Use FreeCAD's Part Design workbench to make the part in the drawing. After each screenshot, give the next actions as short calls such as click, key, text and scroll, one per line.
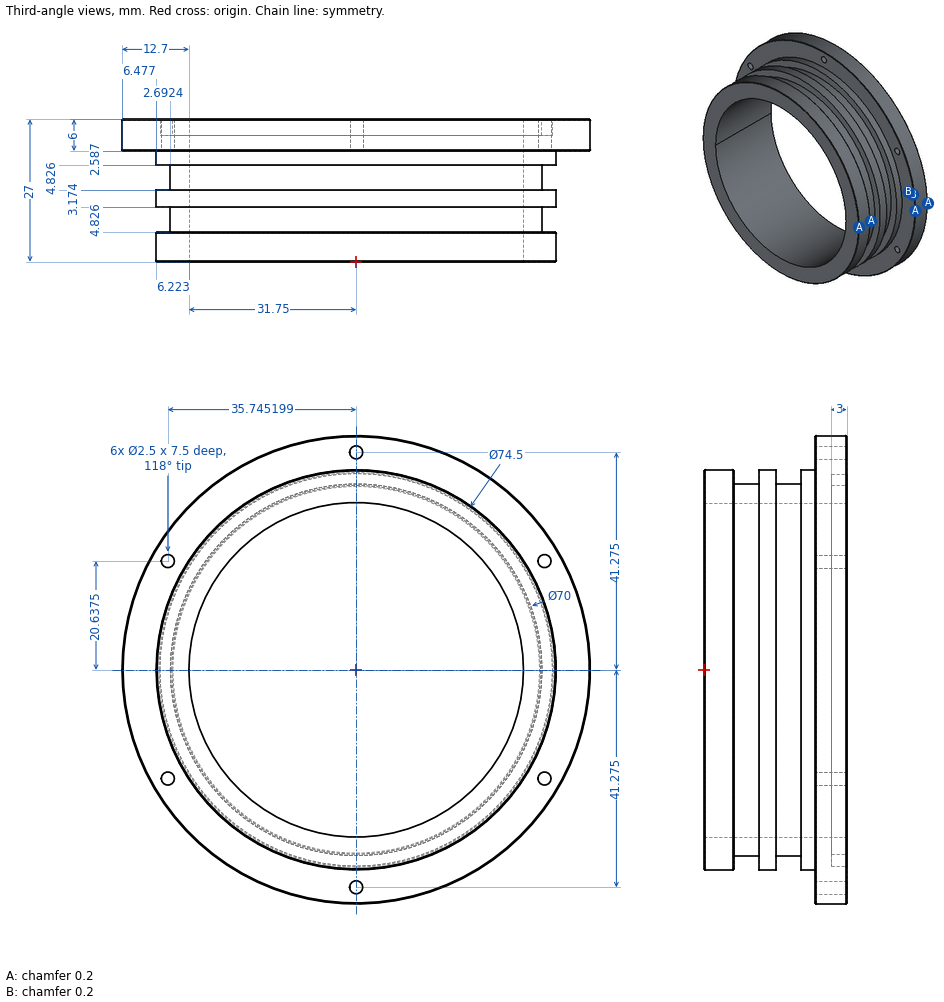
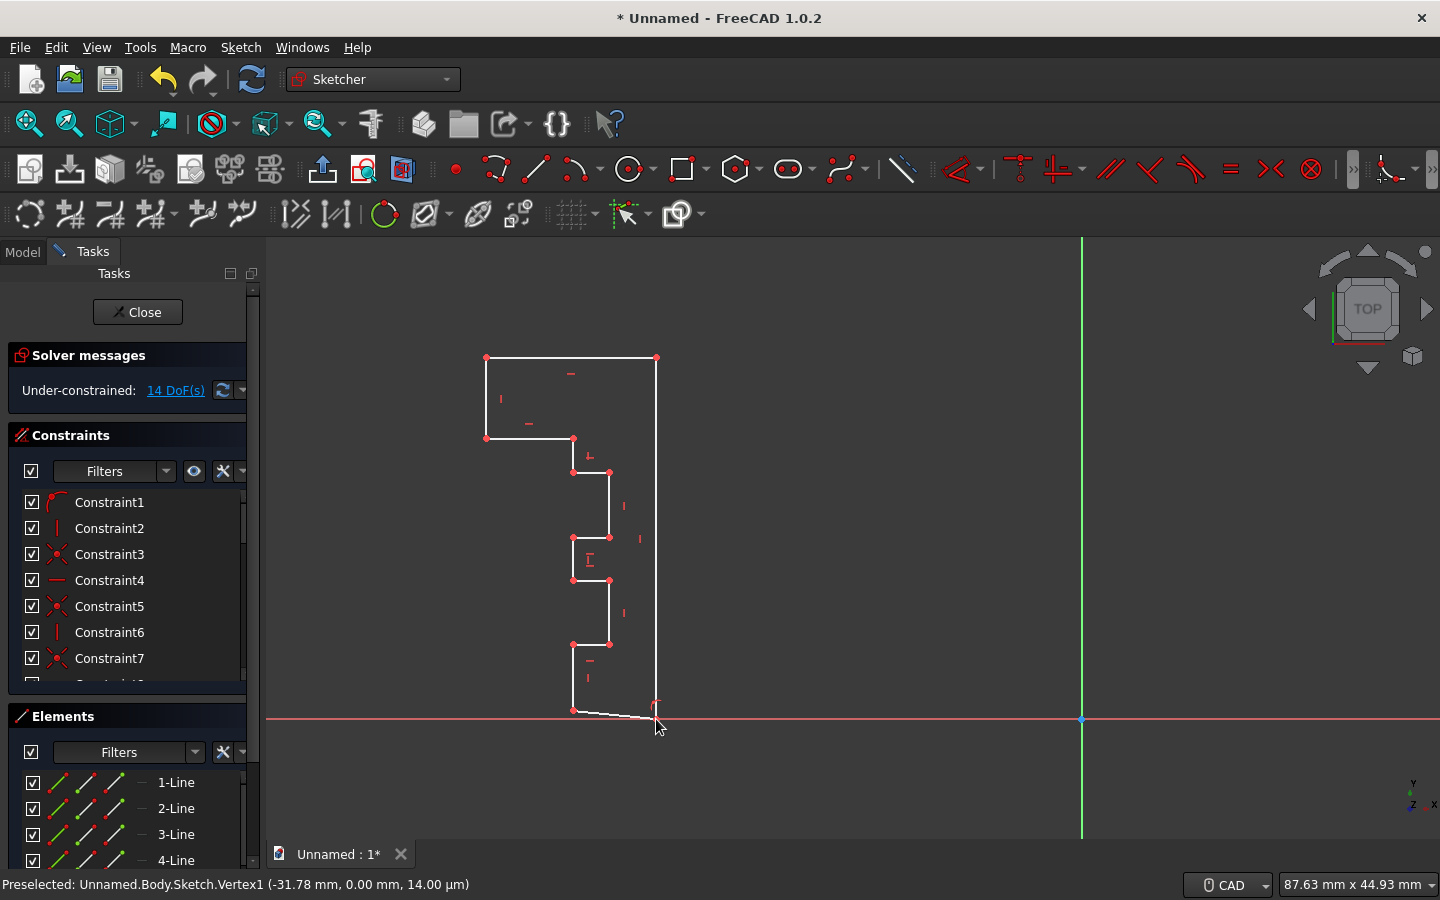
click(631, 717)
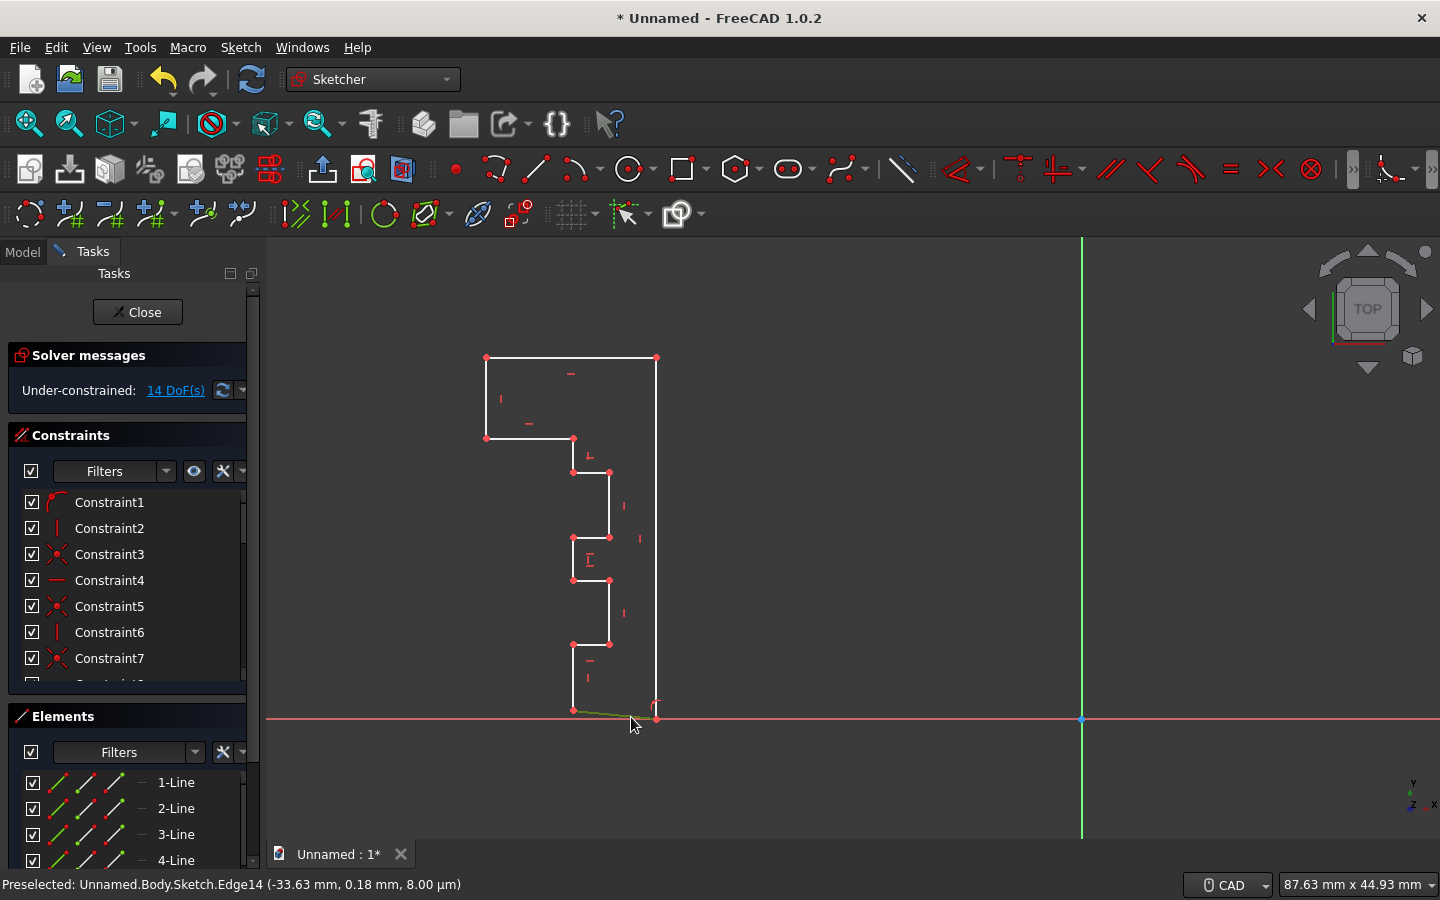
key(h)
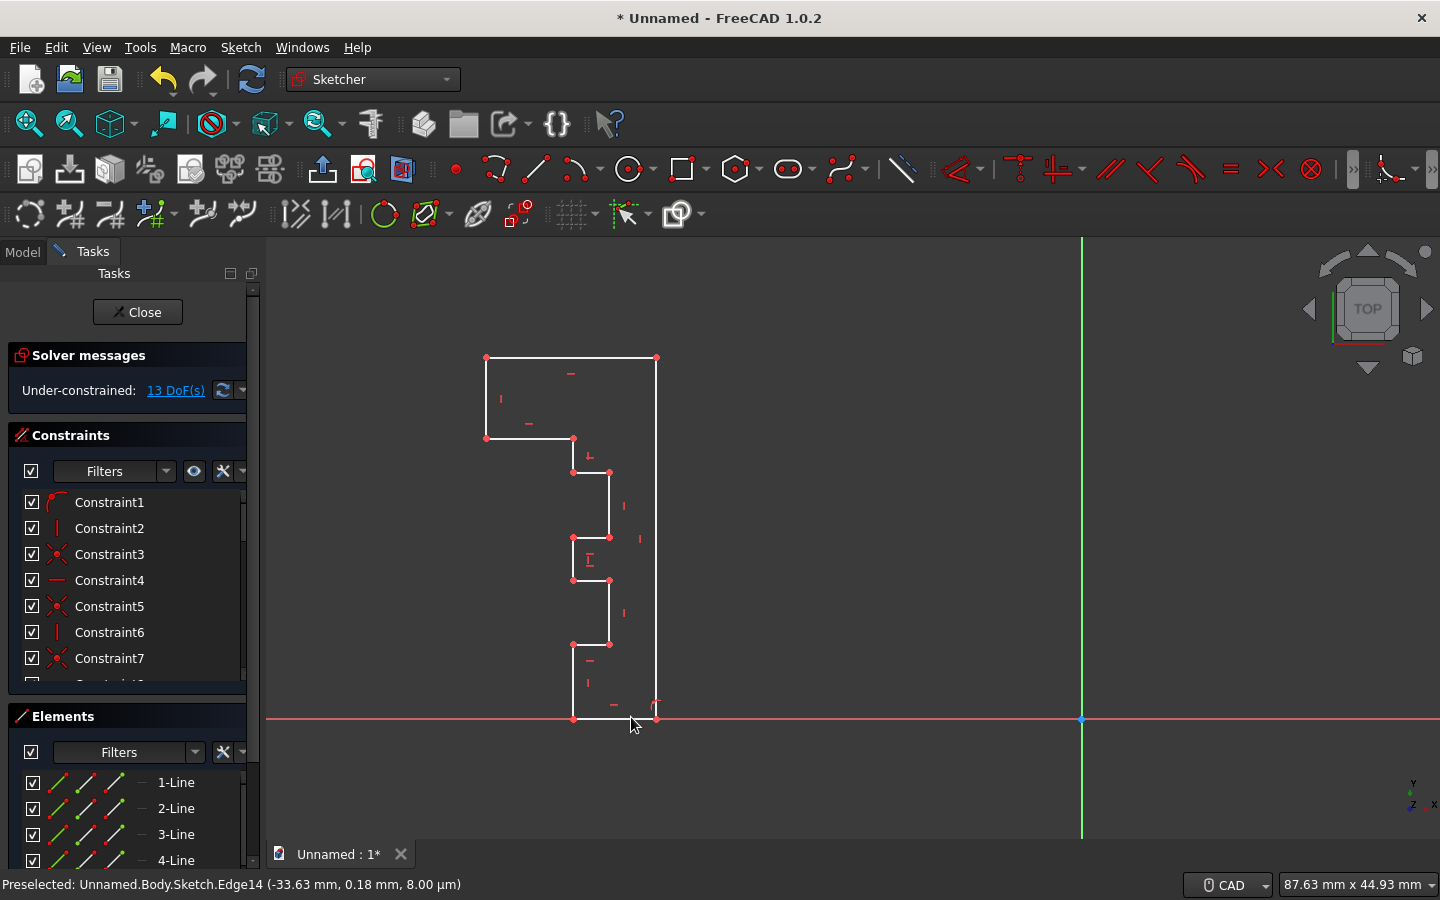
click(486, 382)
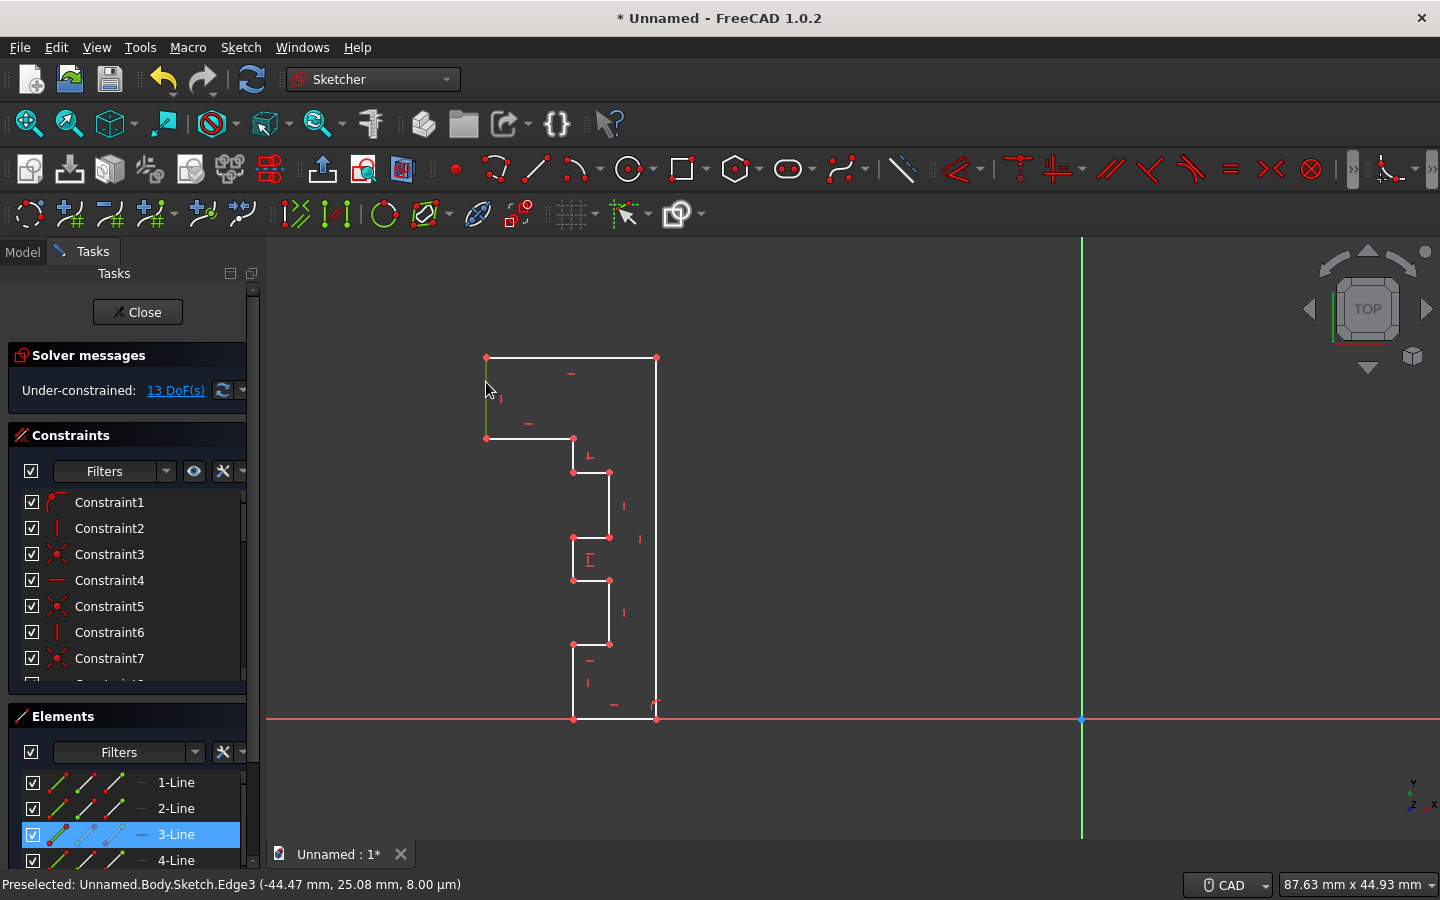
key(i)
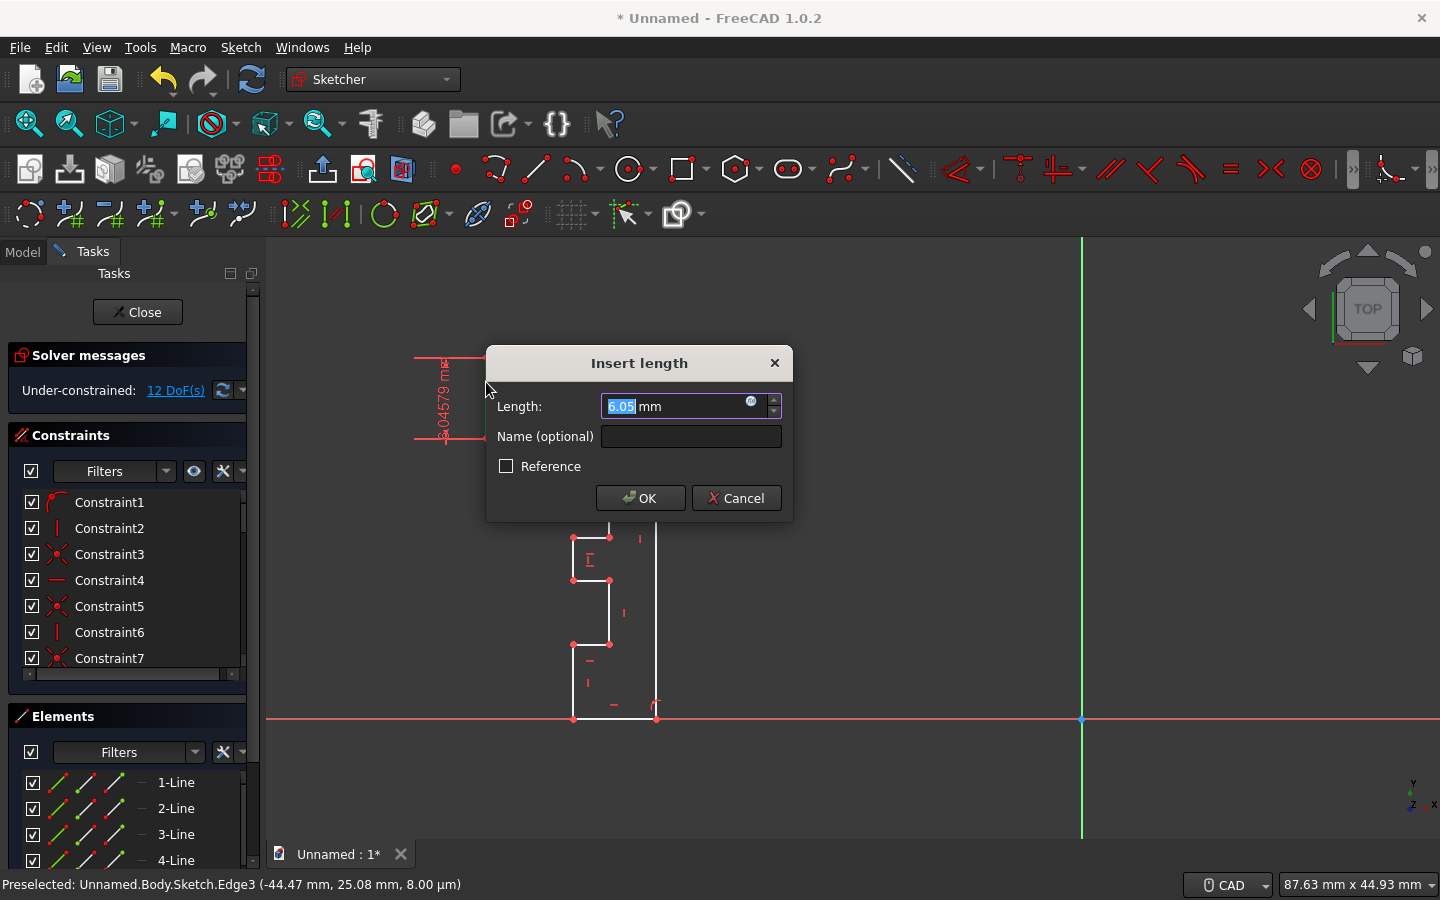
text(6)
key(Return)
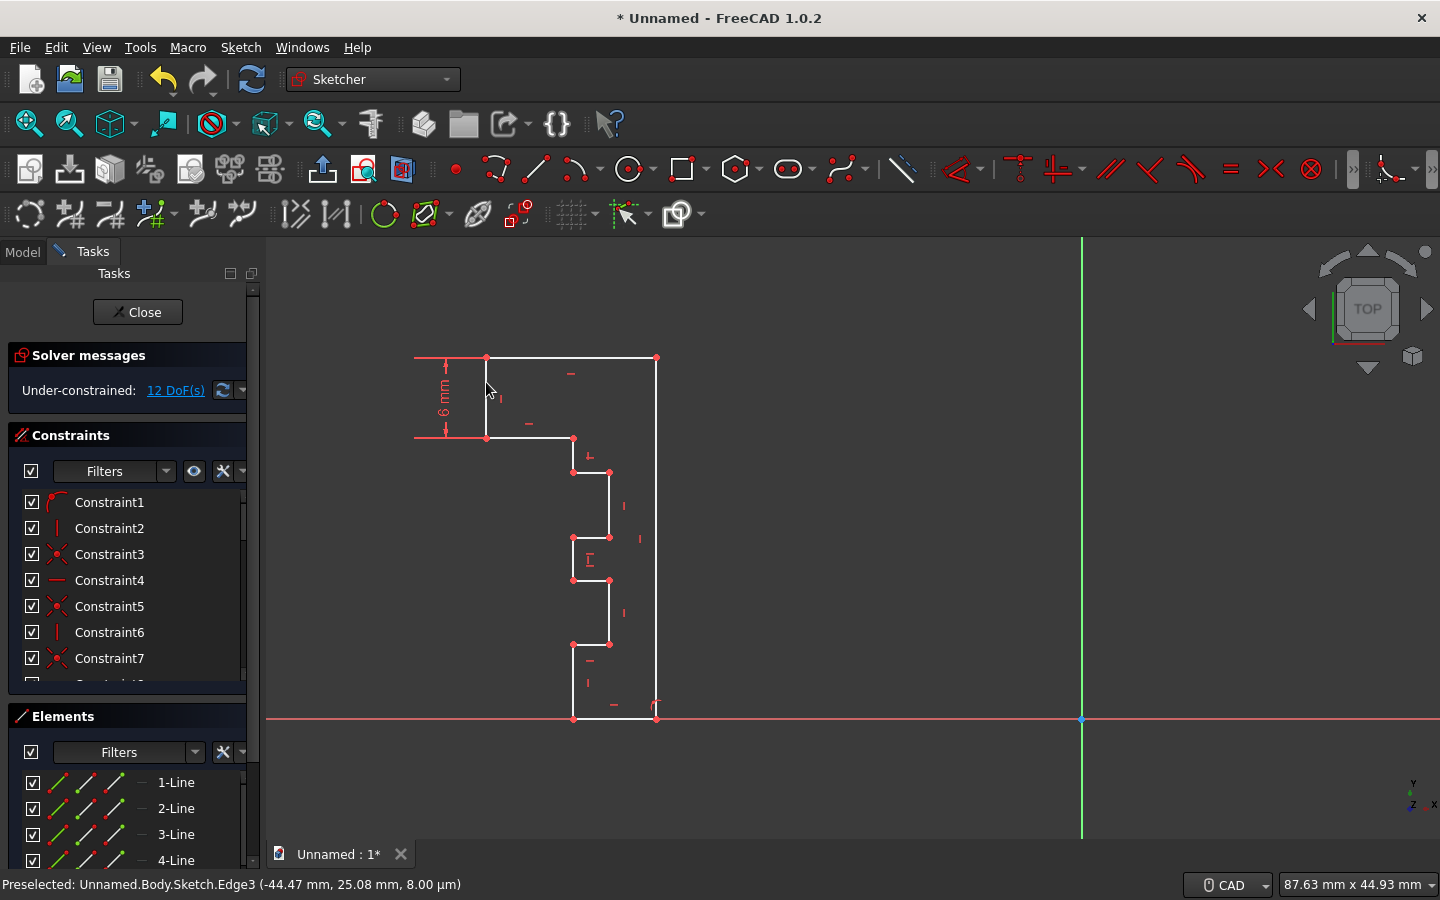
click(656, 611)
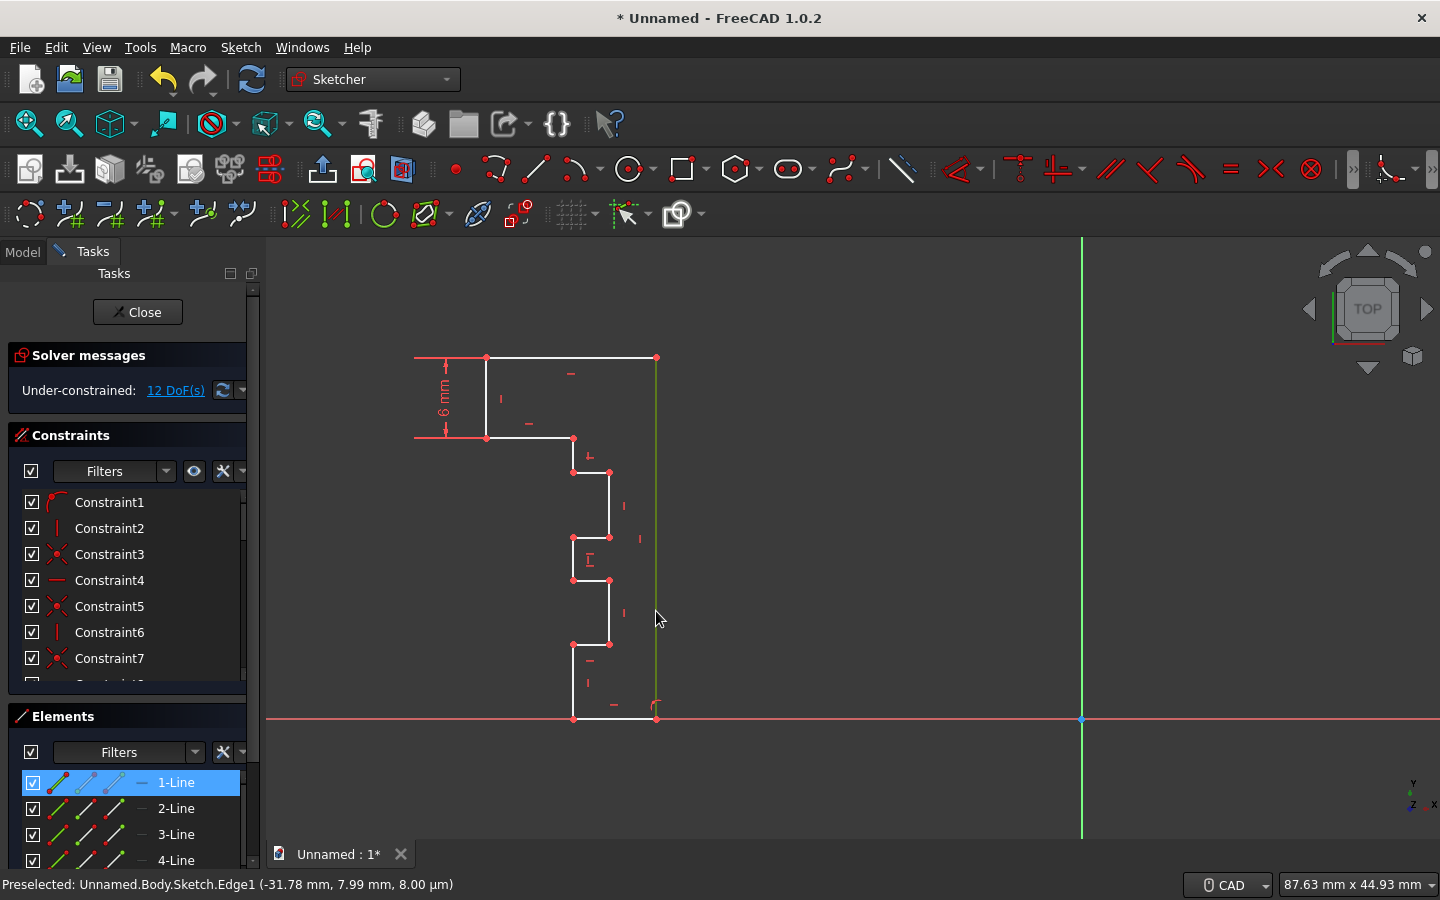
key(i)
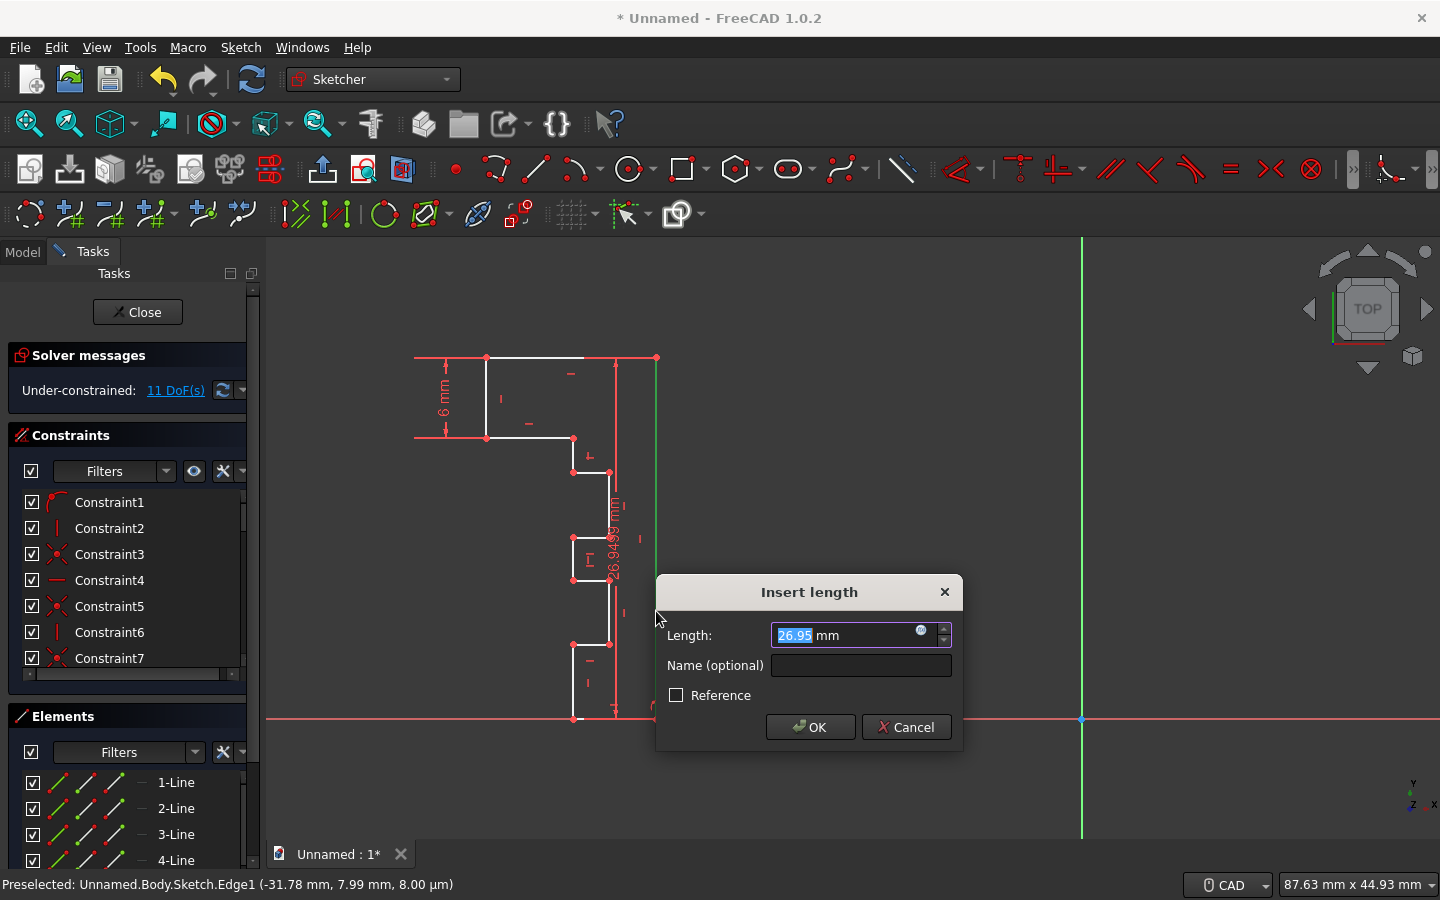
text(27)
key(Return)